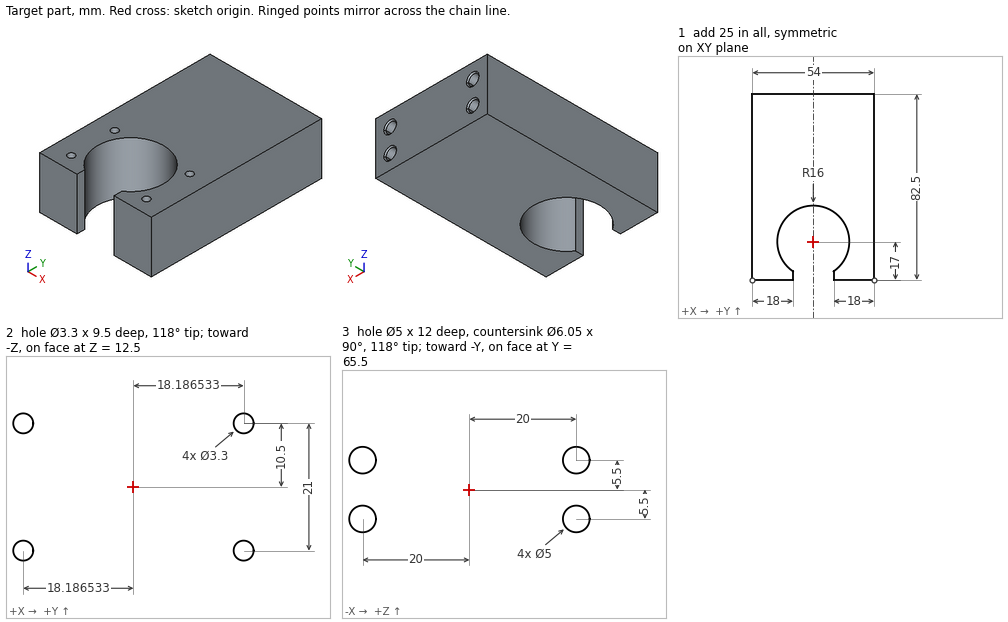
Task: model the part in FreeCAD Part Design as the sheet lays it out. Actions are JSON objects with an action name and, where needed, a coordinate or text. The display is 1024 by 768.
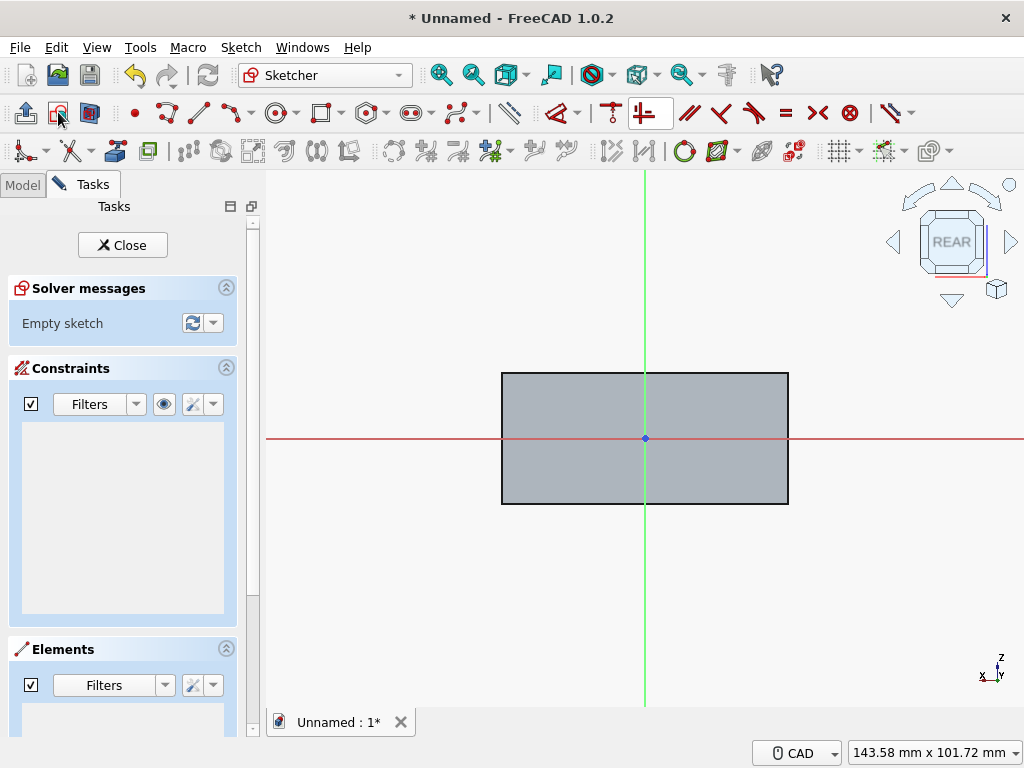
{"action": "scroll", "coordinate": [728, 438], "scroll_direction": "up", "scroll_amount": 3}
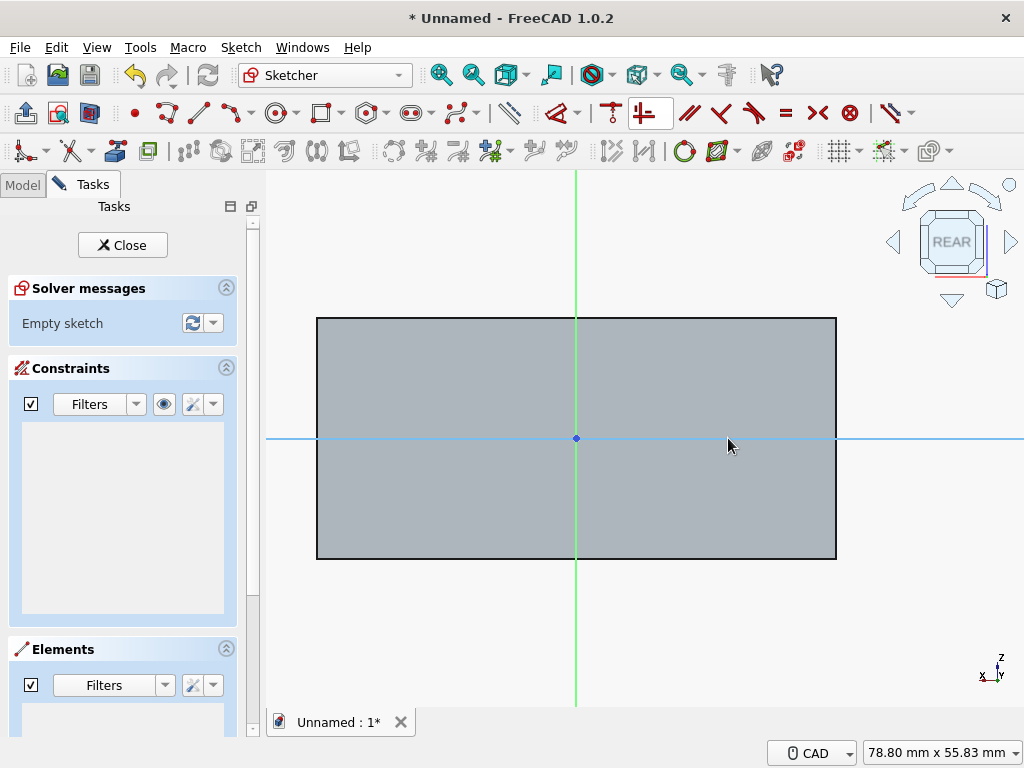
{"action": "left_click", "coordinate": [276, 114]}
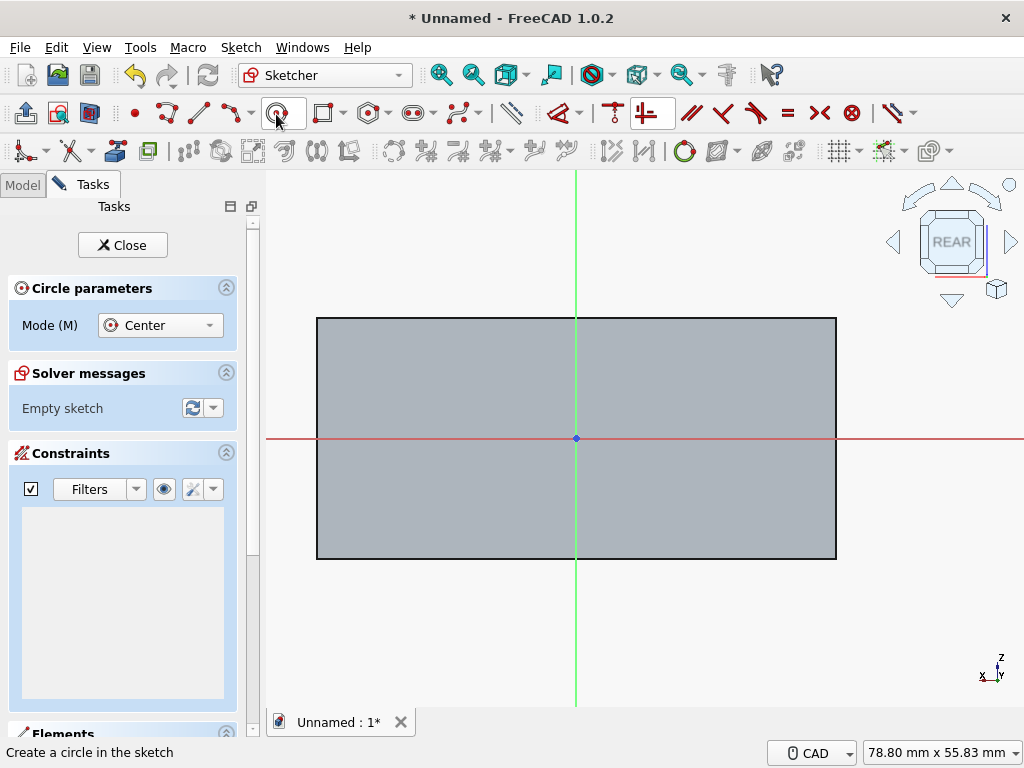
{"action": "left_click", "coordinate": [769, 386]}
{"action": "left_click", "coordinate": [786, 369]}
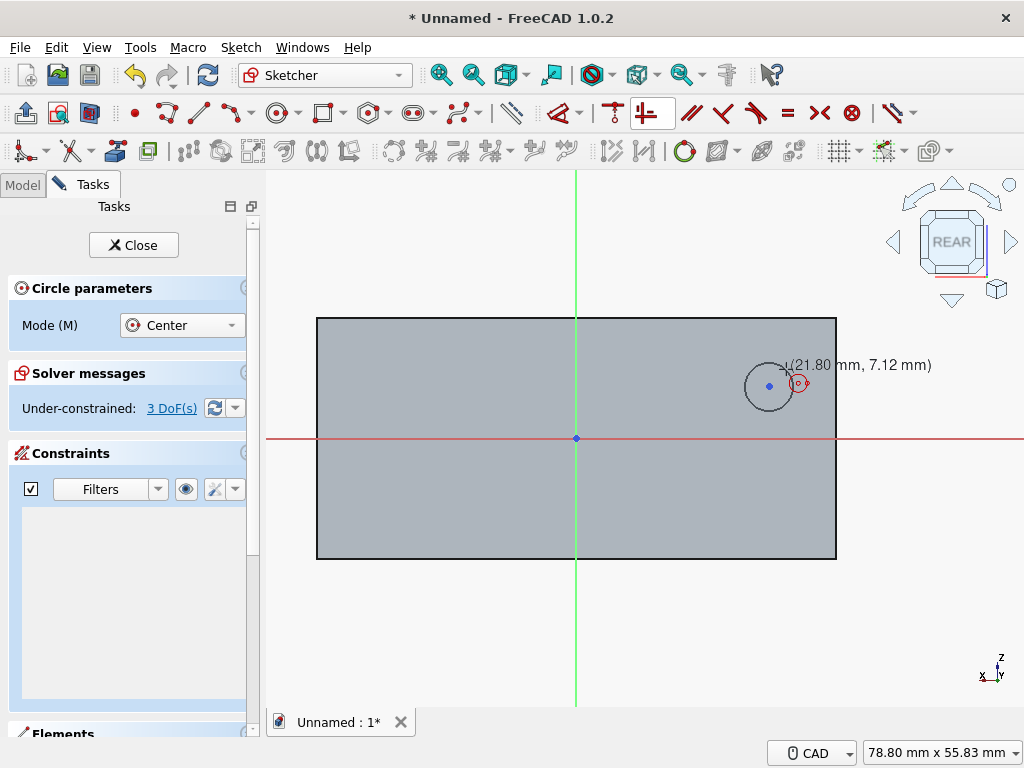
{"action": "left_click", "coordinate": [769, 491]}
{"action": "left_click", "coordinate": [786, 474]}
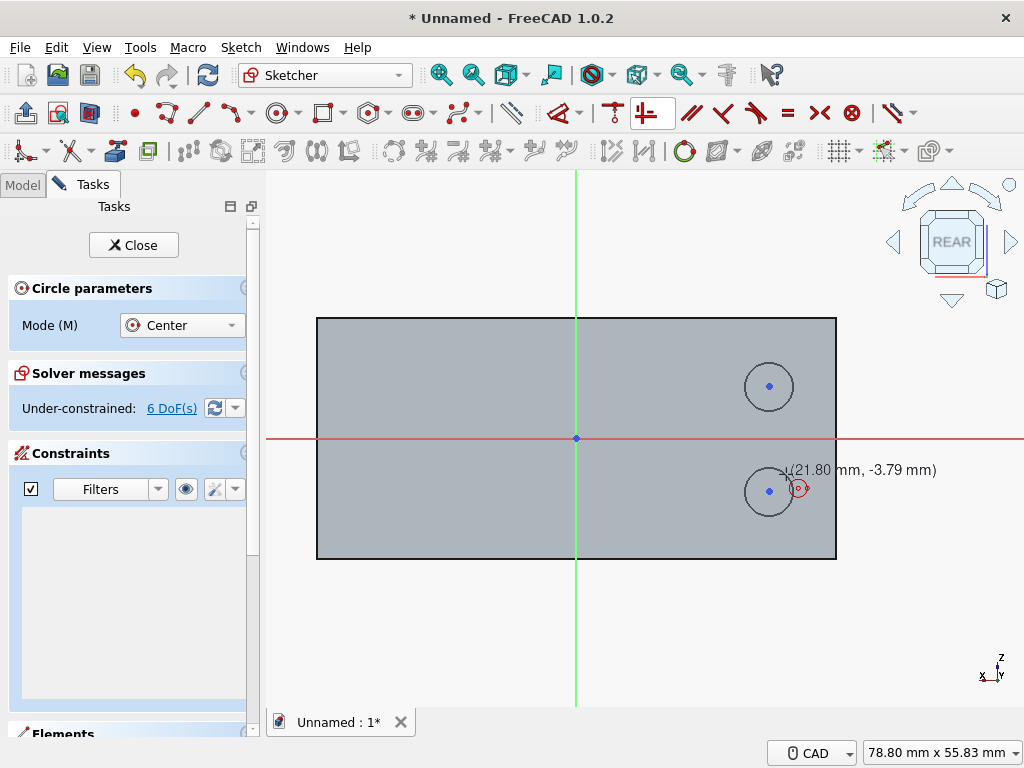
{"action": "left_click", "coordinate": [384, 491]}
{"action": "left_click", "coordinate": [401, 474]}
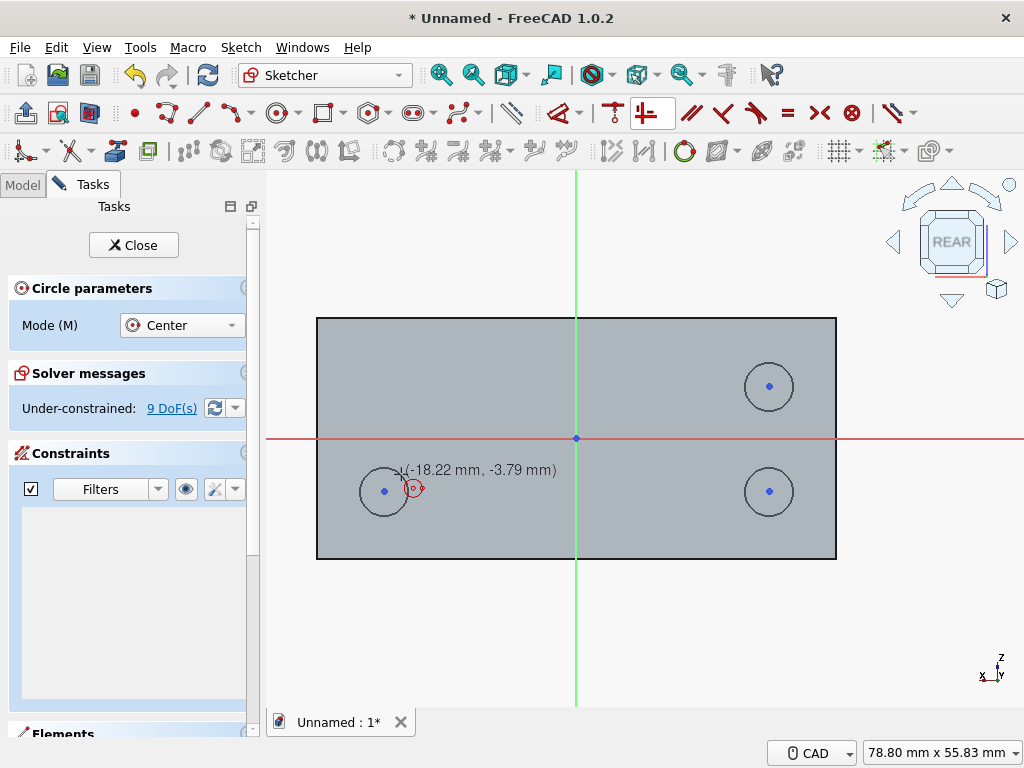
{"action": "left_click", "coordinate": [384, 386]}
{"action": "left_click", "coordinate": [401, 369]}
{"action": "key", "text": "Escape"}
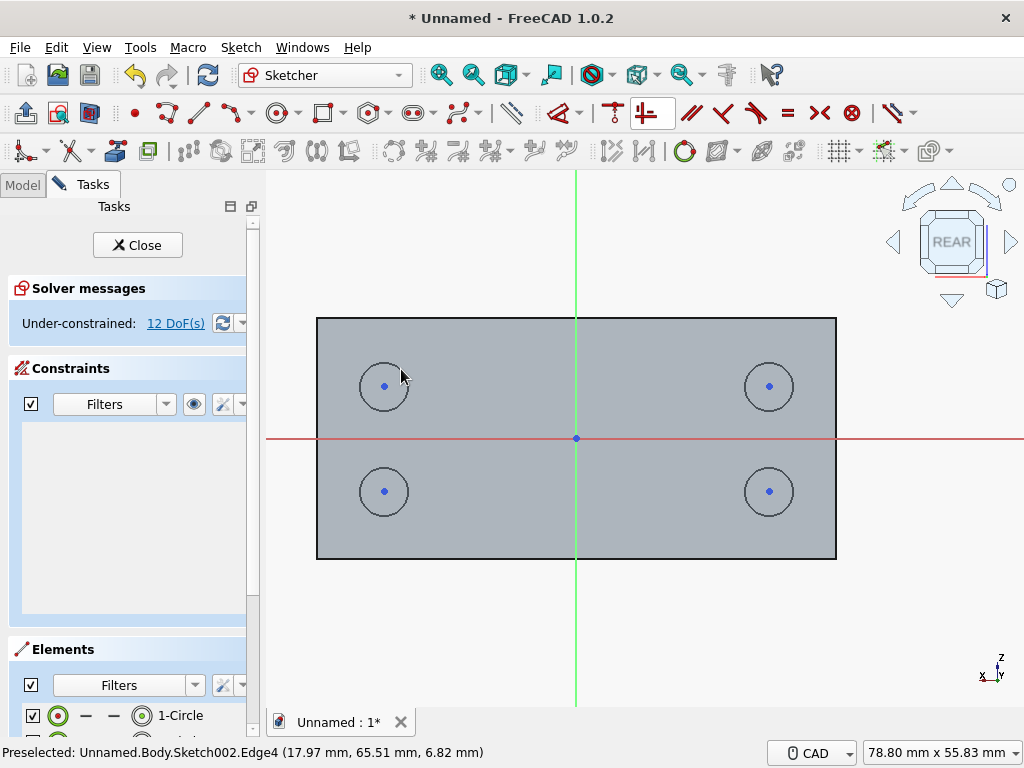
{"action": "left_click", "coordinate": [786, 370]}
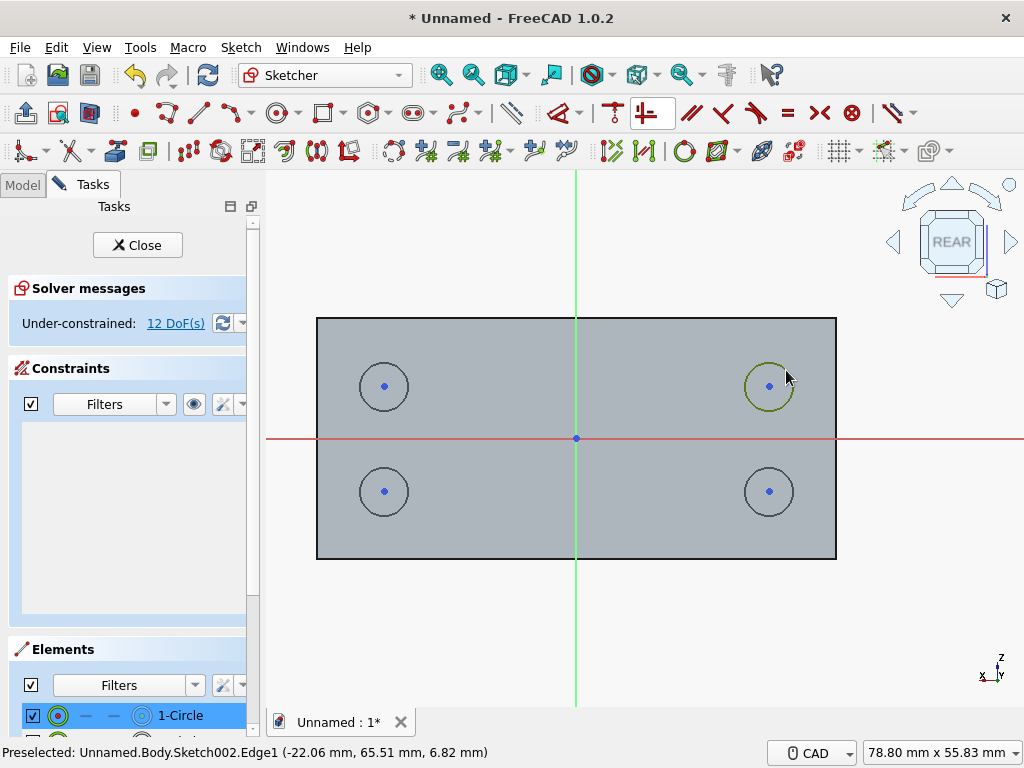
{"action": "left_click", "coordinate": [786, 475]}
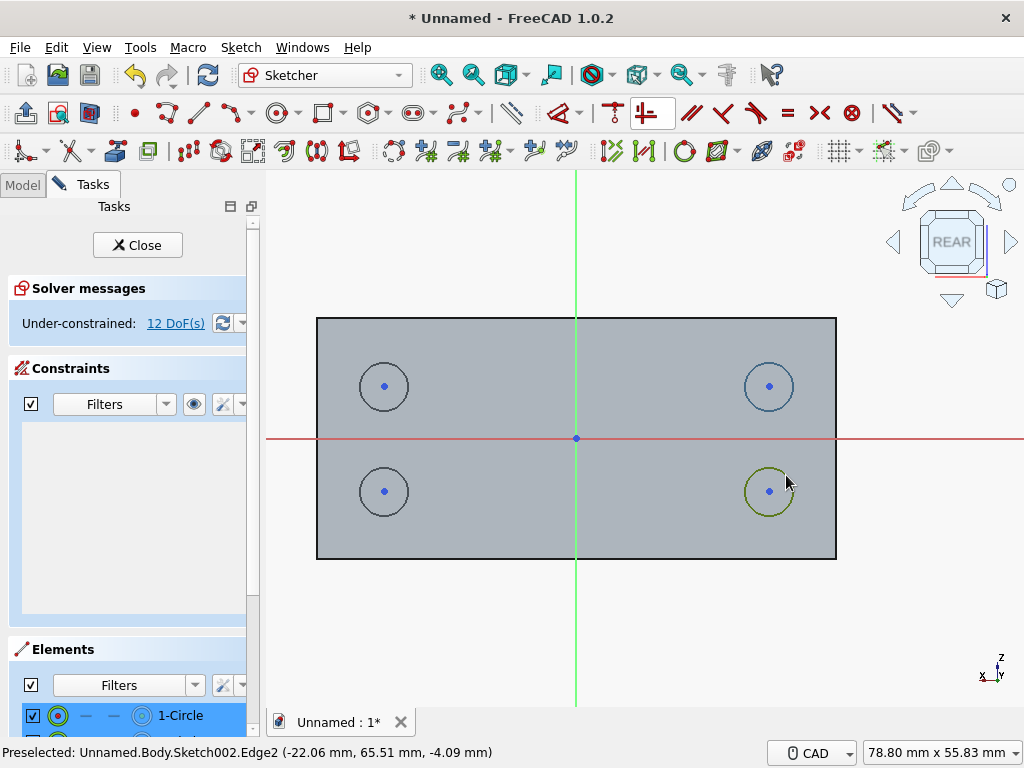
{"action": "left_click", "coordinate": [401, 475]}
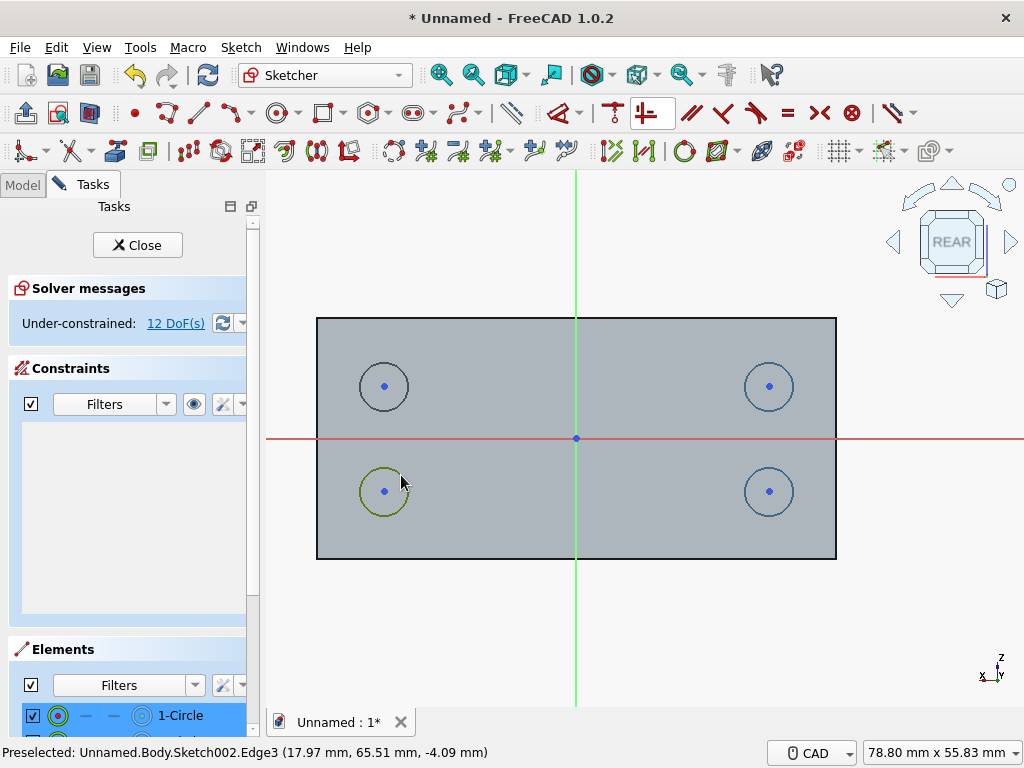
{"action": "left_click", "coordinate": [401, 370]}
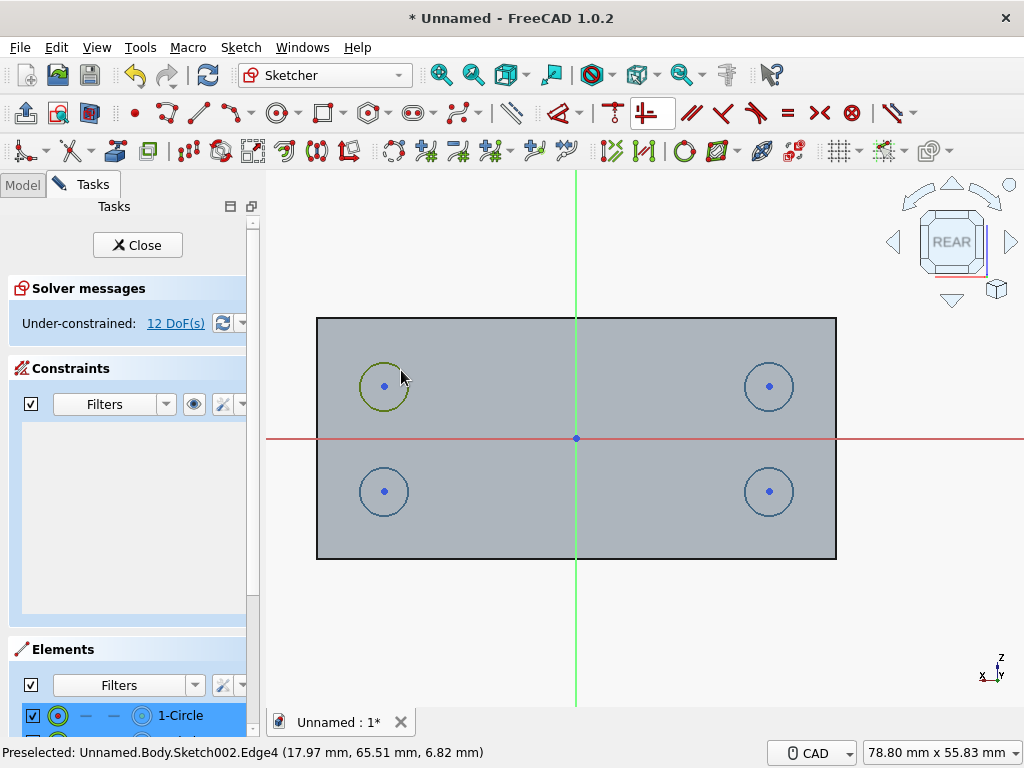
{"action": "left_click", "coordinate": [788, 114]}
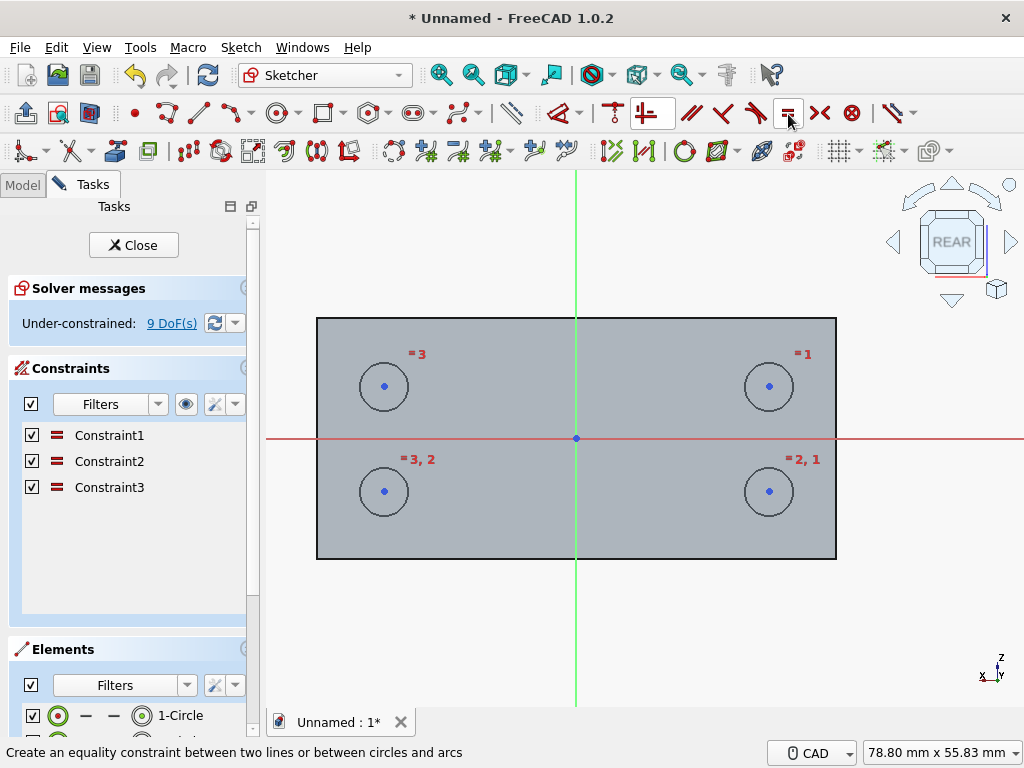
{"action": "left_click", "coordinate": [769, 387]}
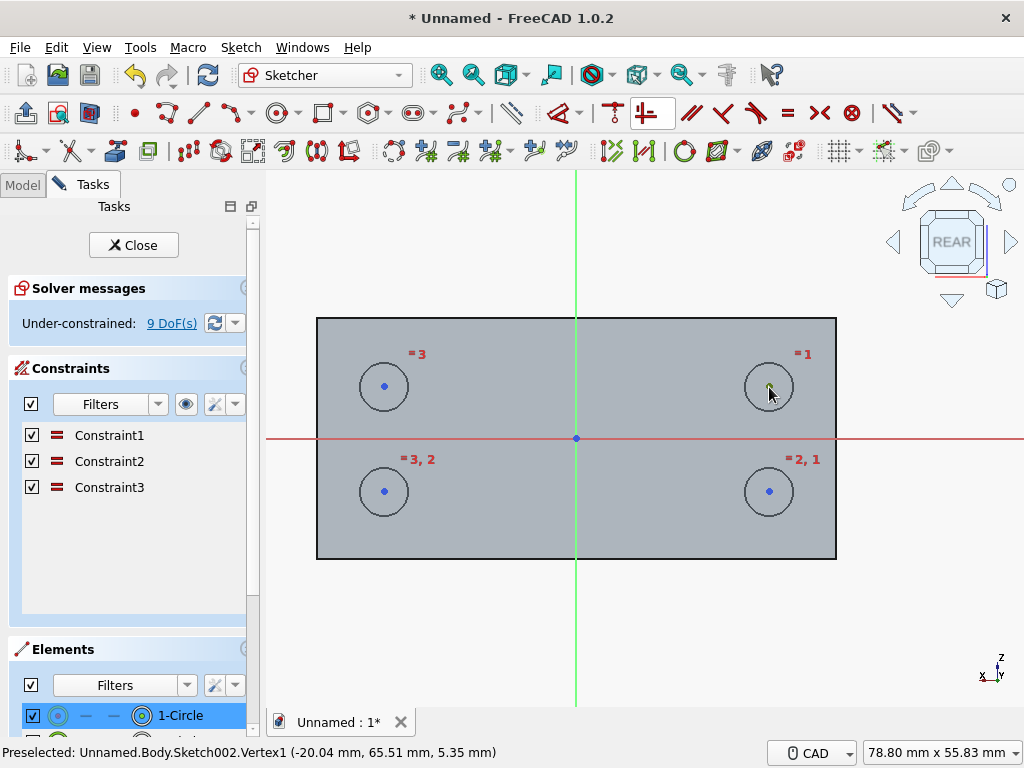
{"action": "left_click", "coordinate": [769, 492]}